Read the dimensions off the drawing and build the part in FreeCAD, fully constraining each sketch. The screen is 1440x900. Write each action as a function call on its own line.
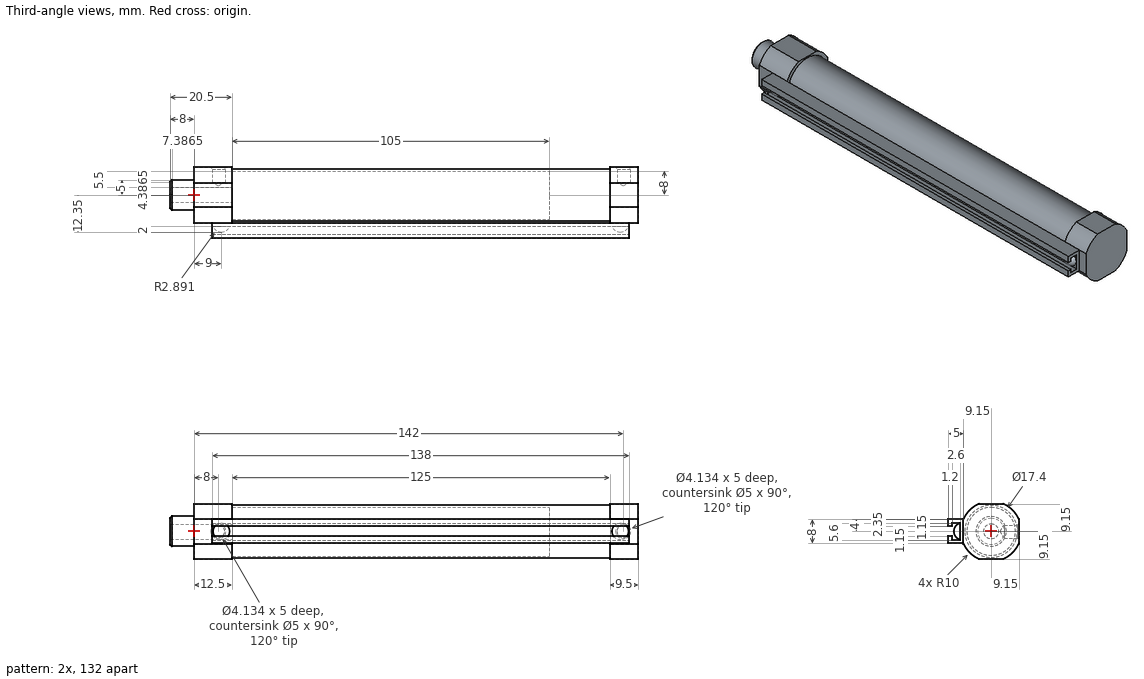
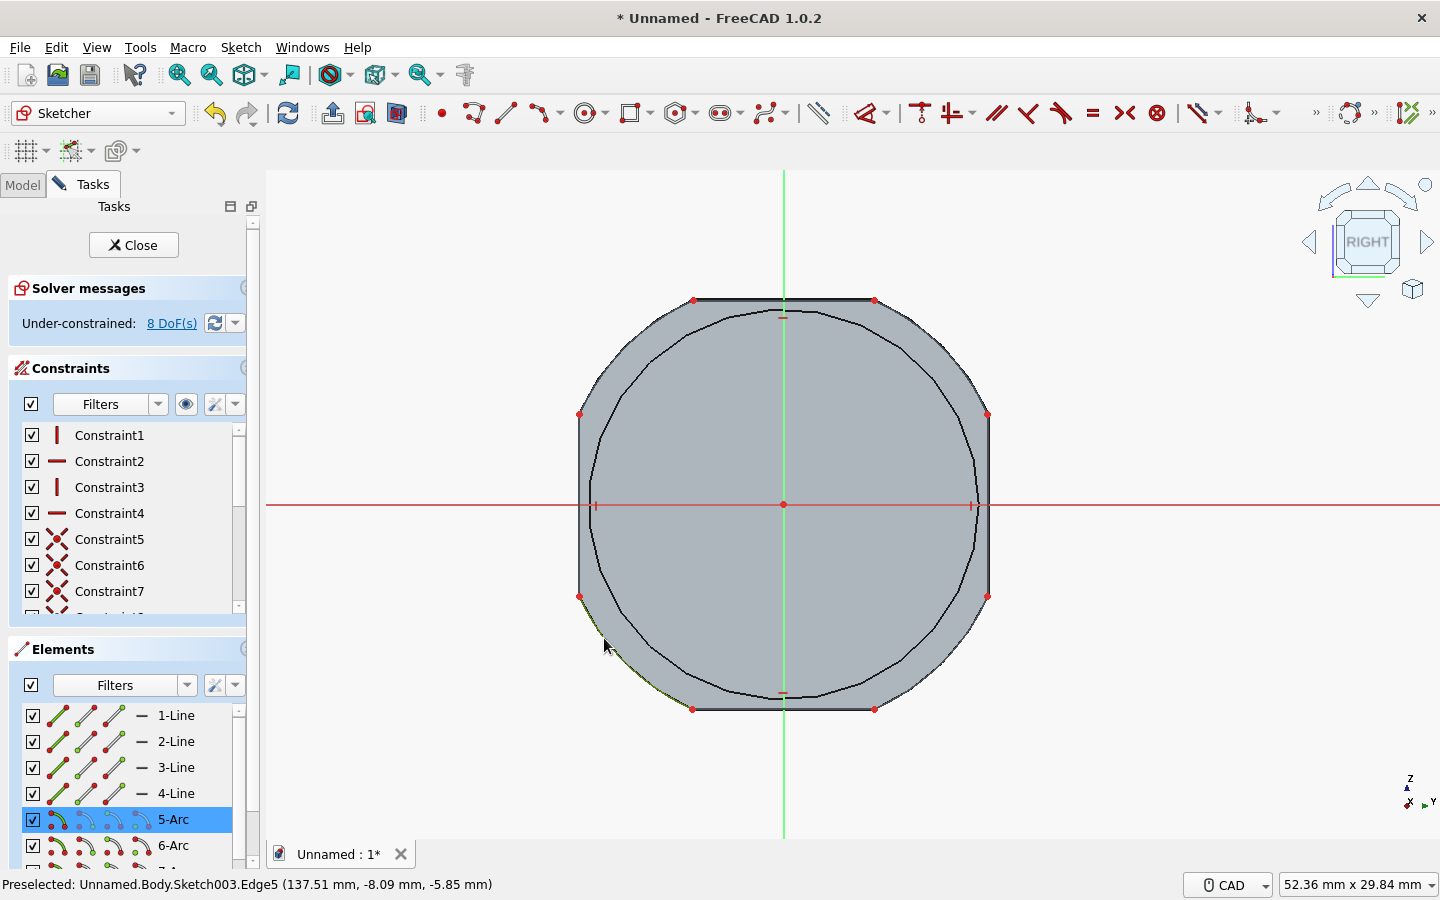
click(917, 684)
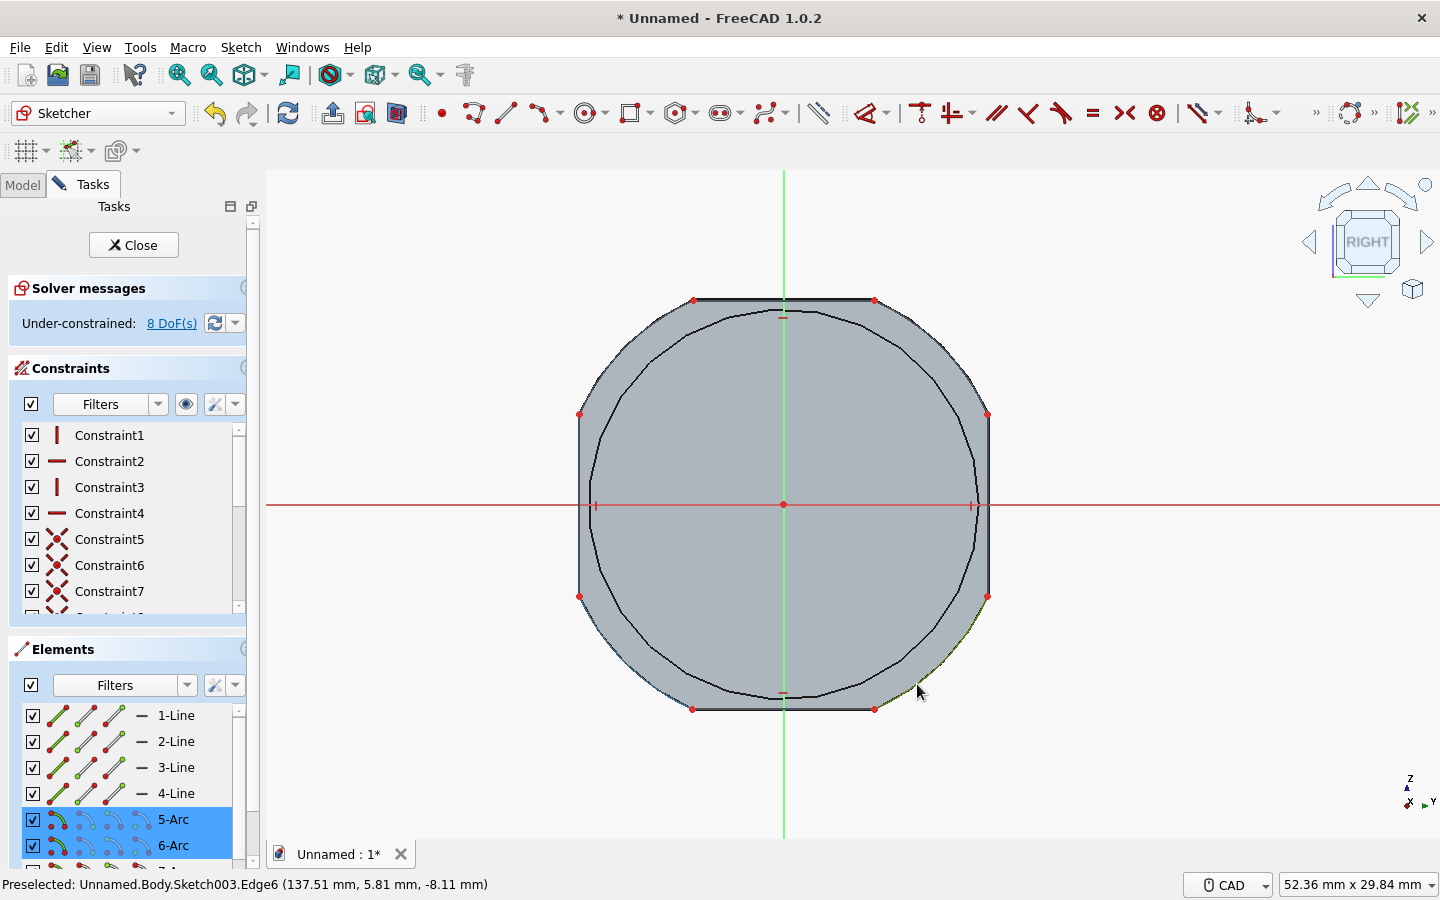
click(963, 372)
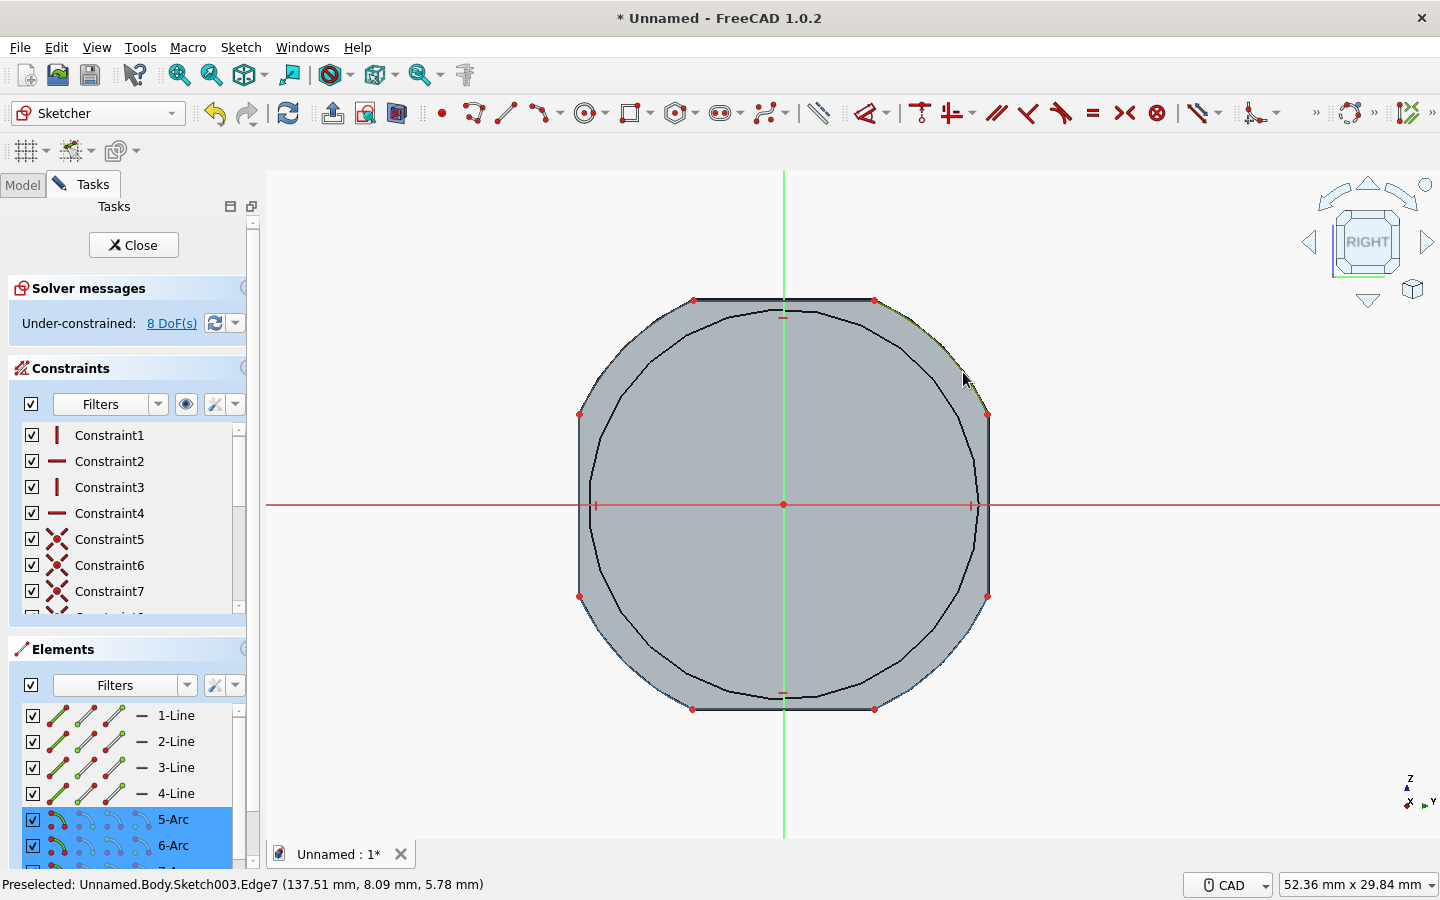
click(650, 326)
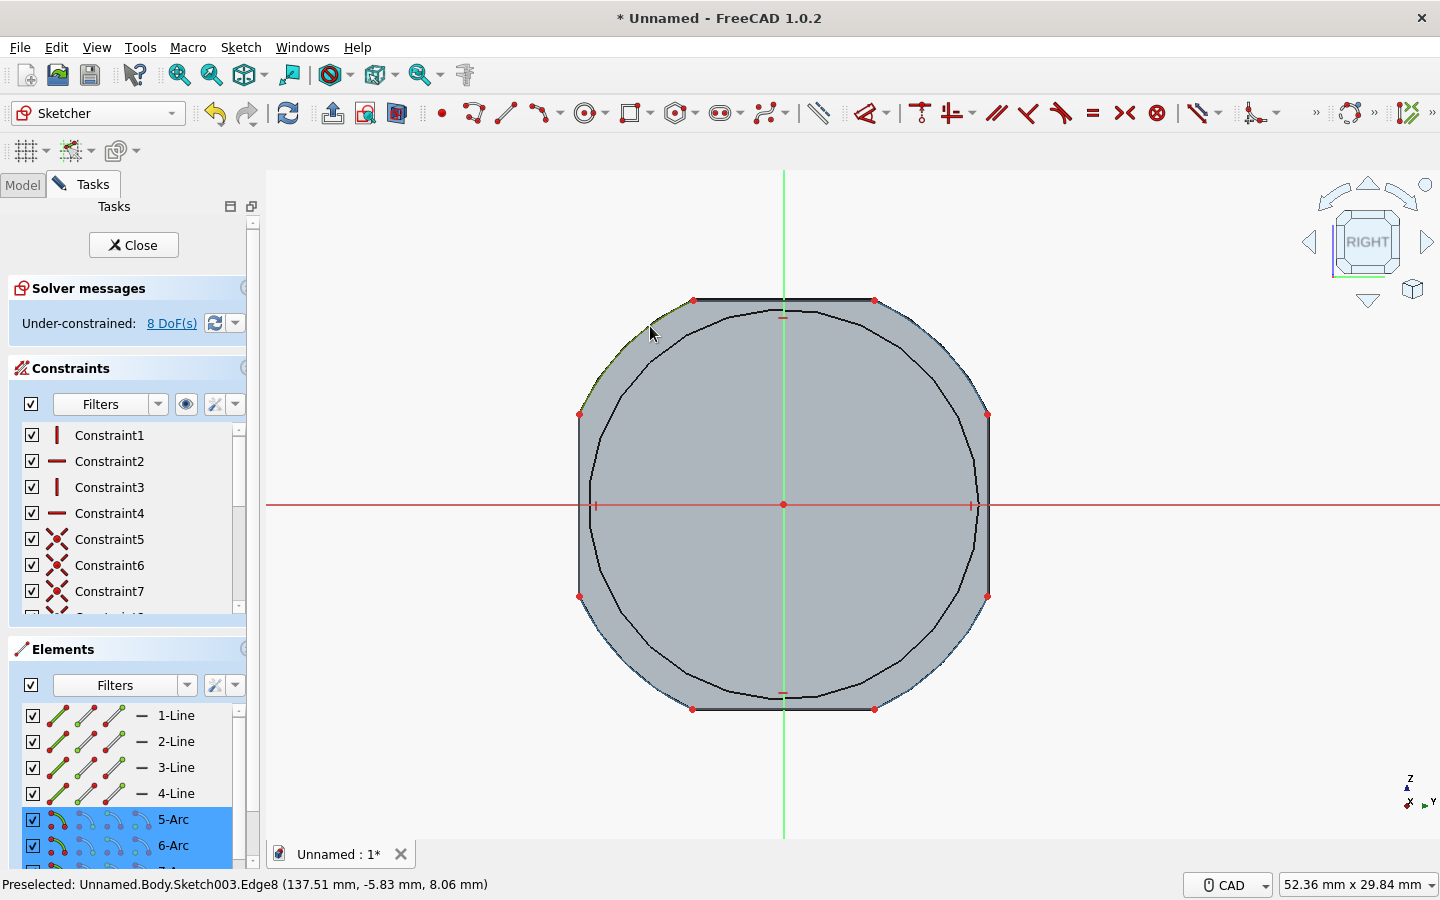
click(1094, 114)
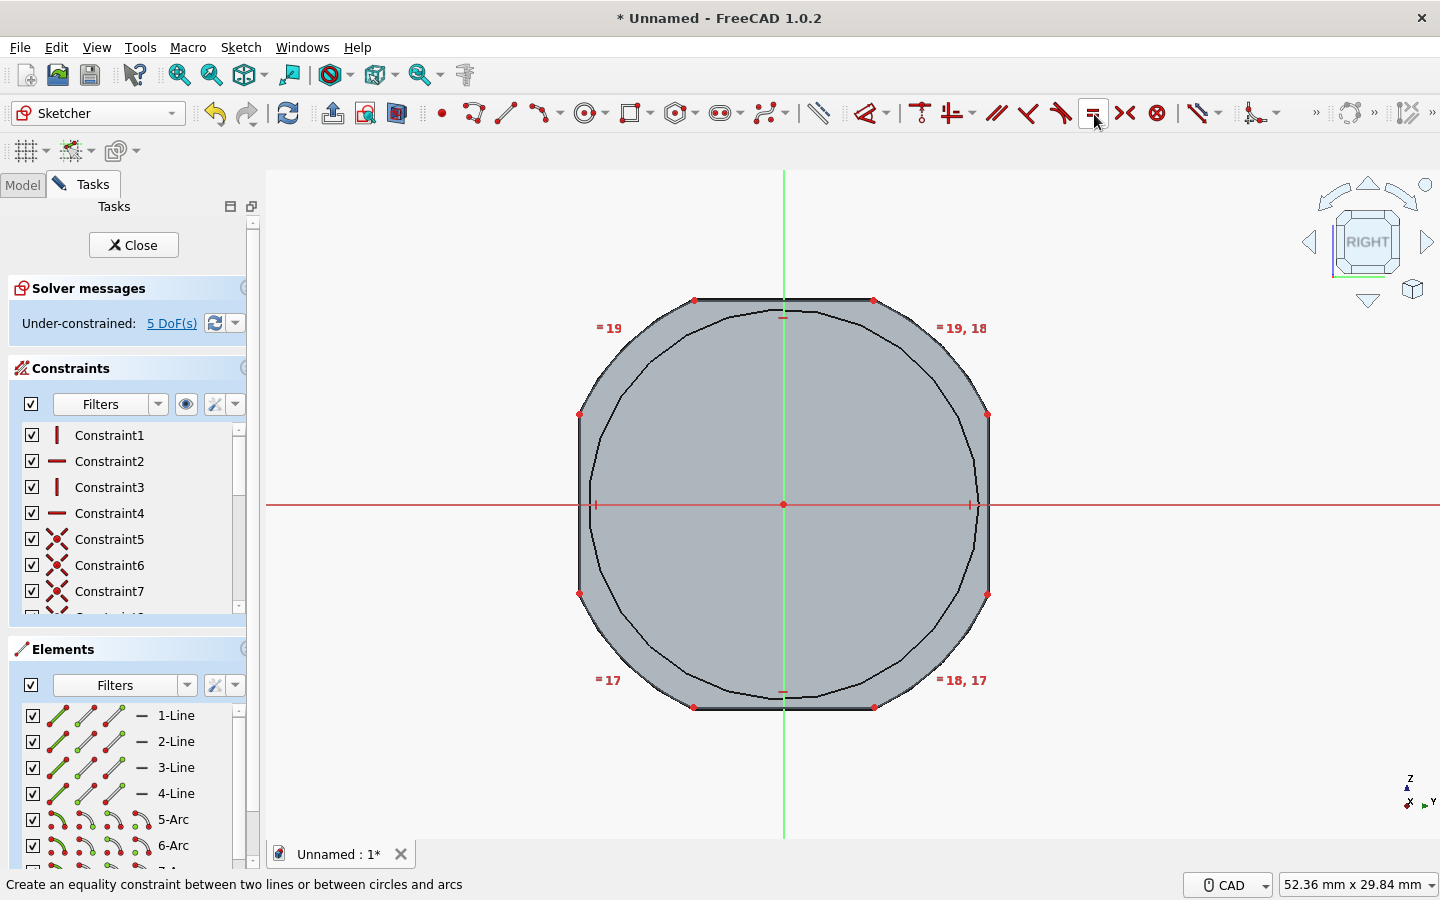
click(866, 114)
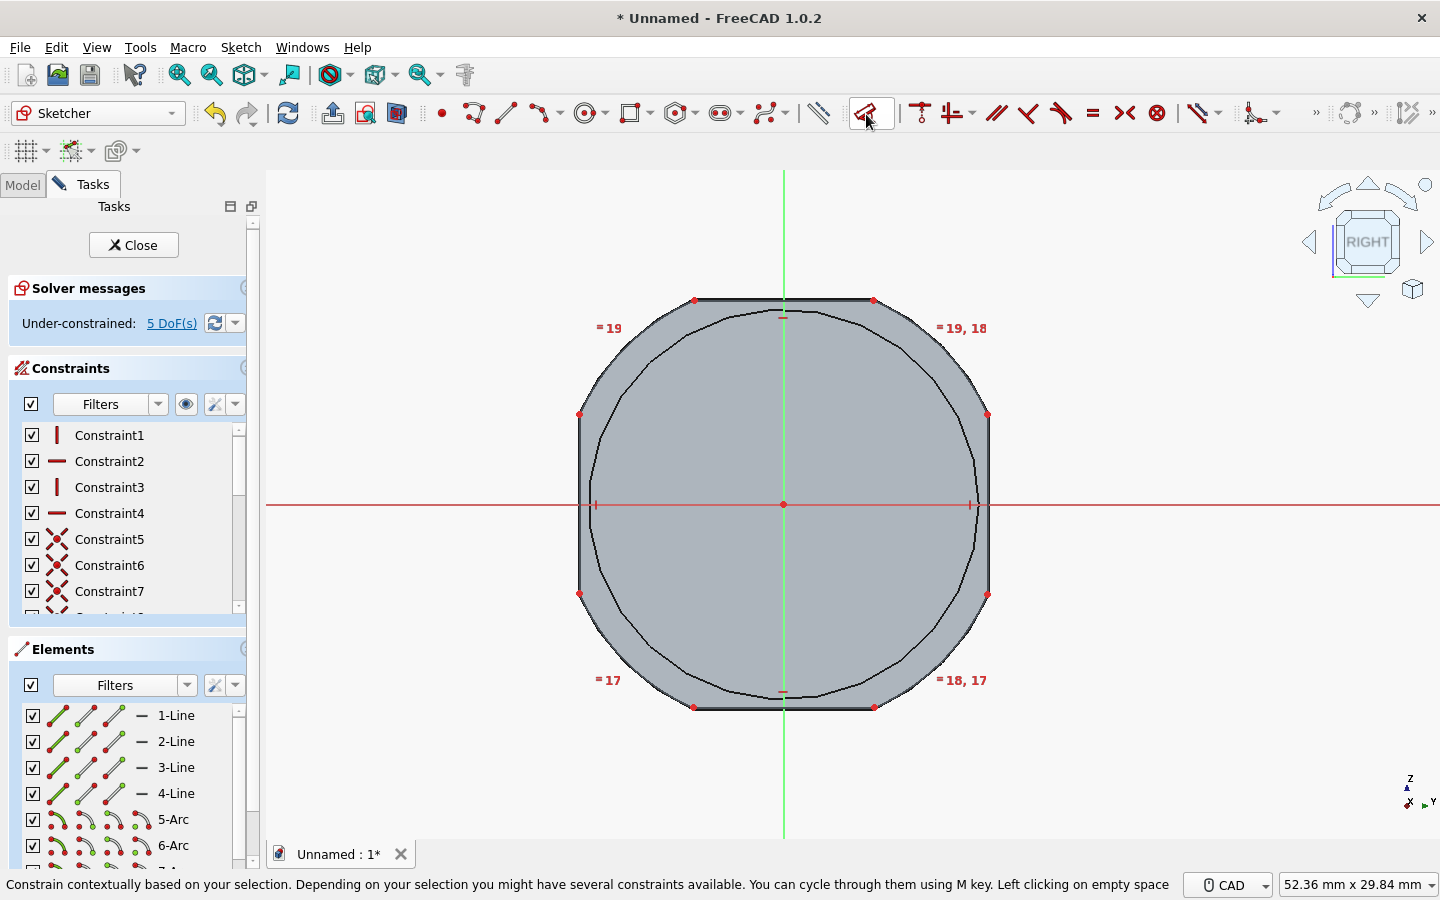
click(605, 637)
click(579, 656)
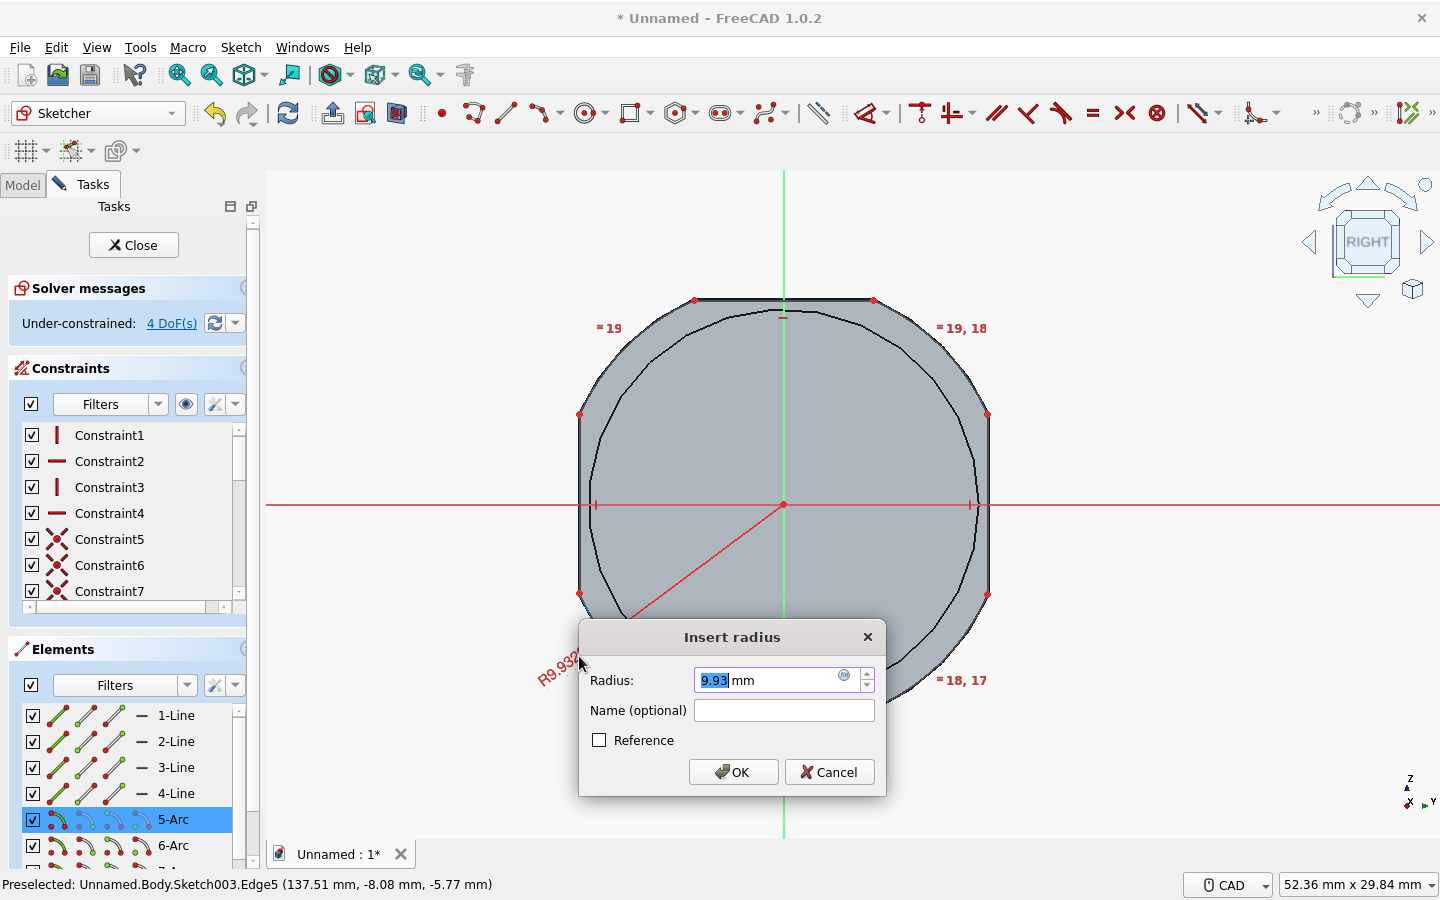
text(10)
key(Return)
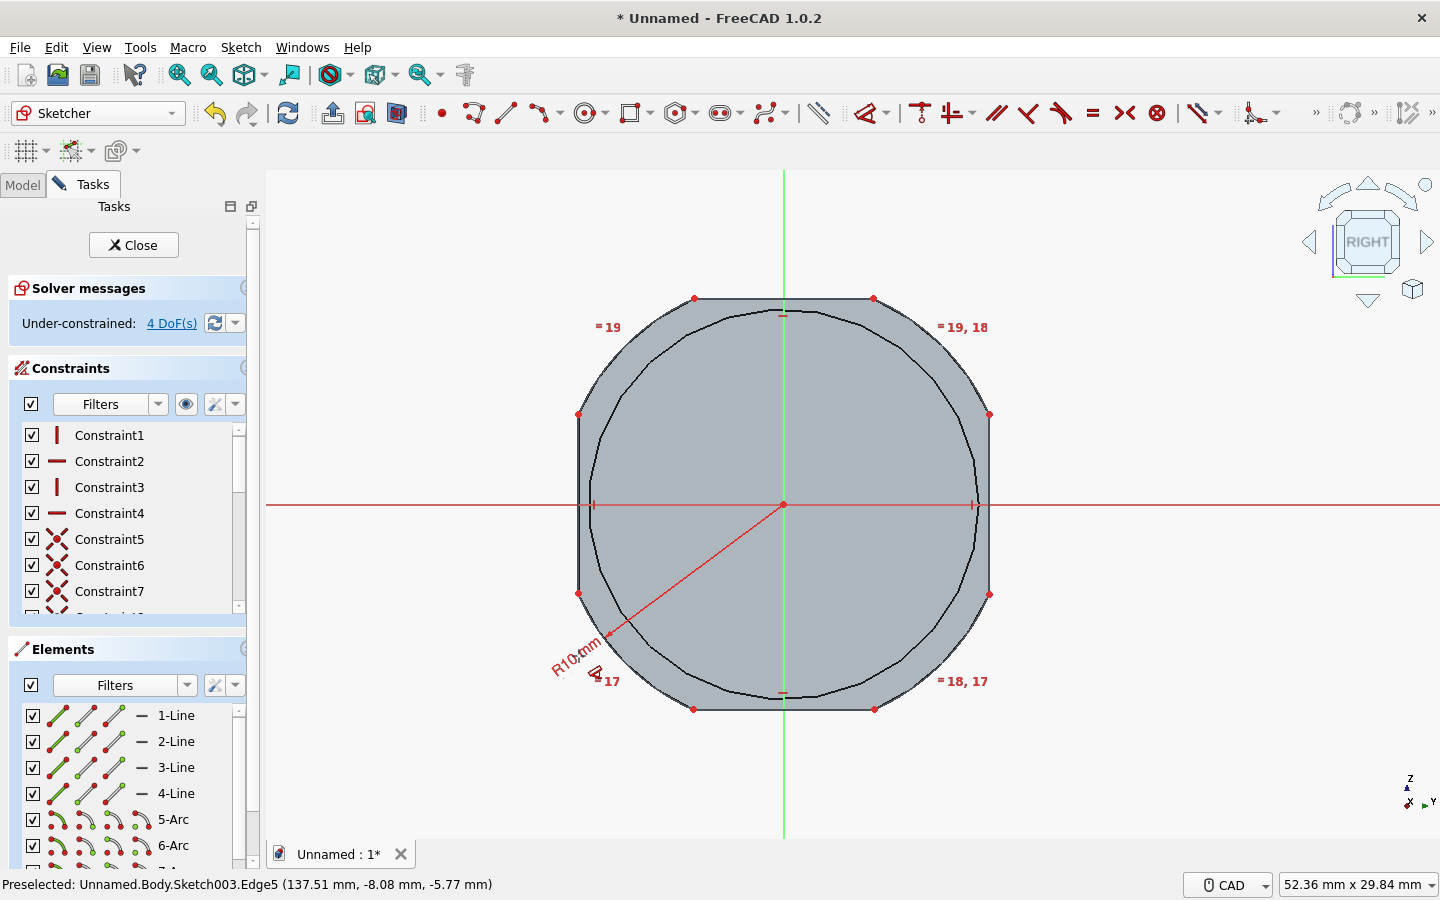
click(578, 415)
click(681, 381)